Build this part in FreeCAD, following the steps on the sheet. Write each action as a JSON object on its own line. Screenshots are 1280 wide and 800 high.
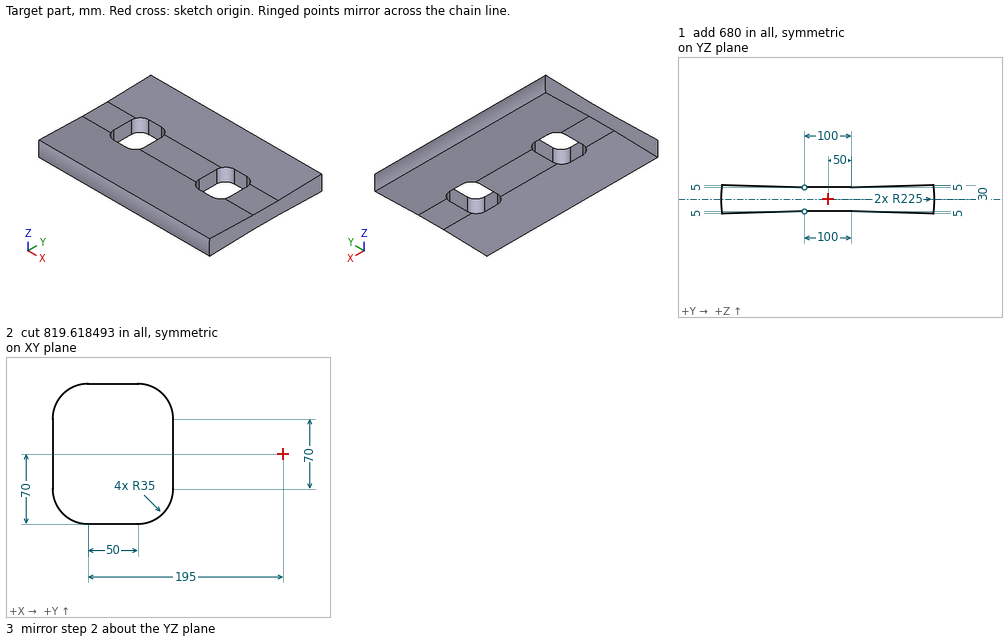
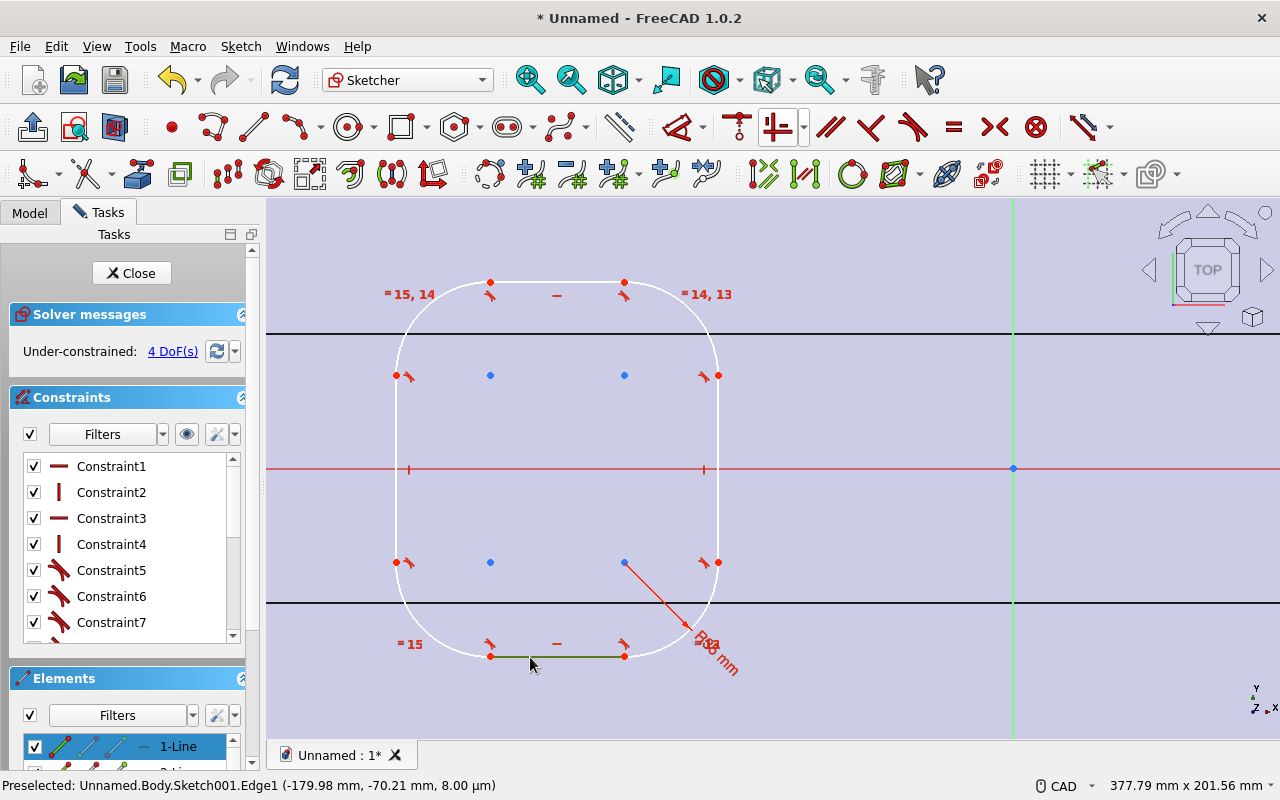
{"action": "key", "text": "l"}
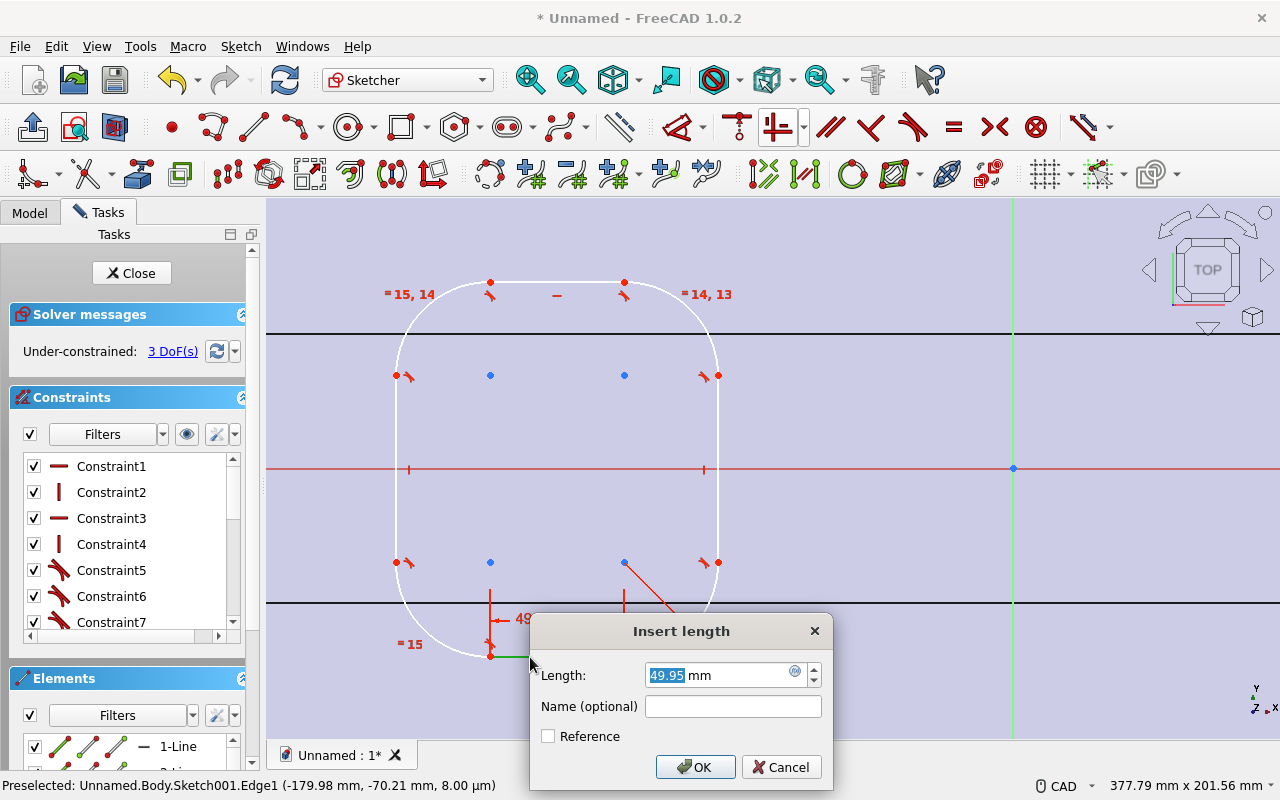
{"action": "type", "text": "50"}
{"action": "key", "text": "Return"}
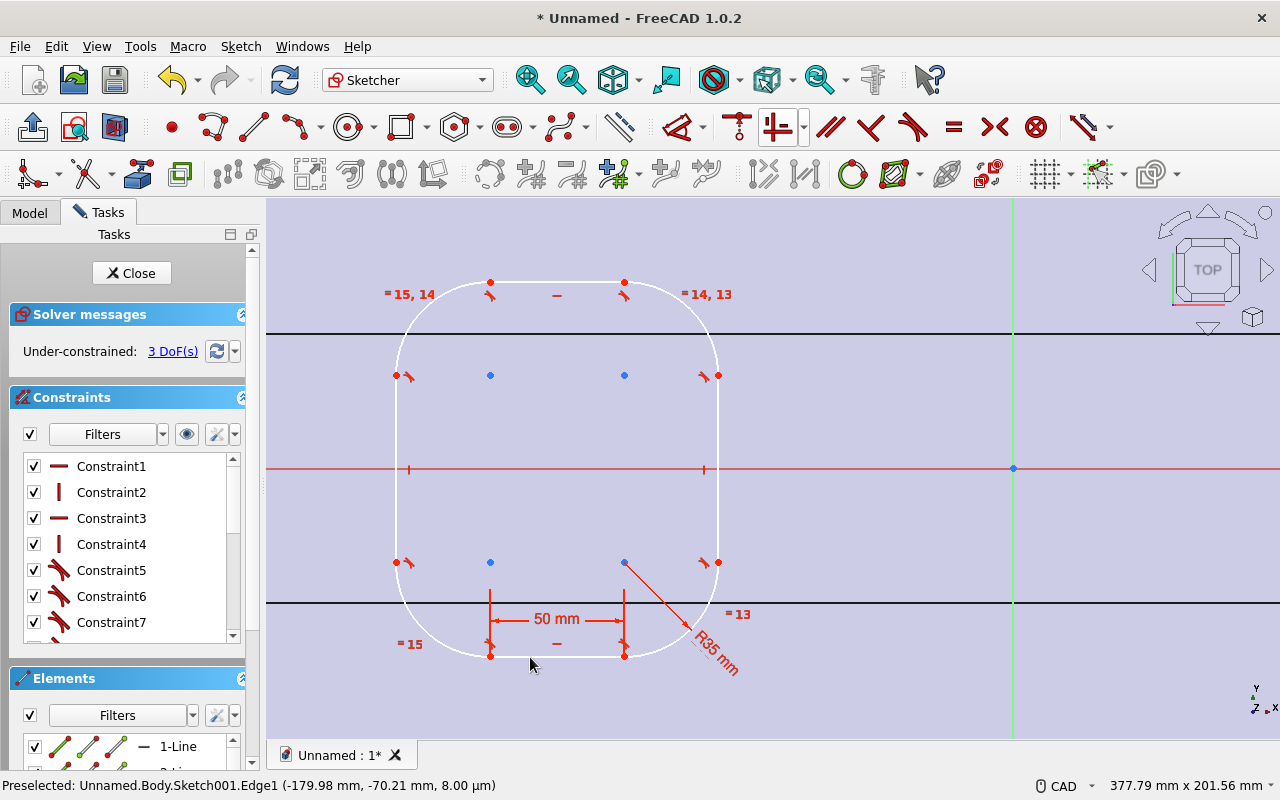
{"action": "left_click", "coordinate": [718, 507]}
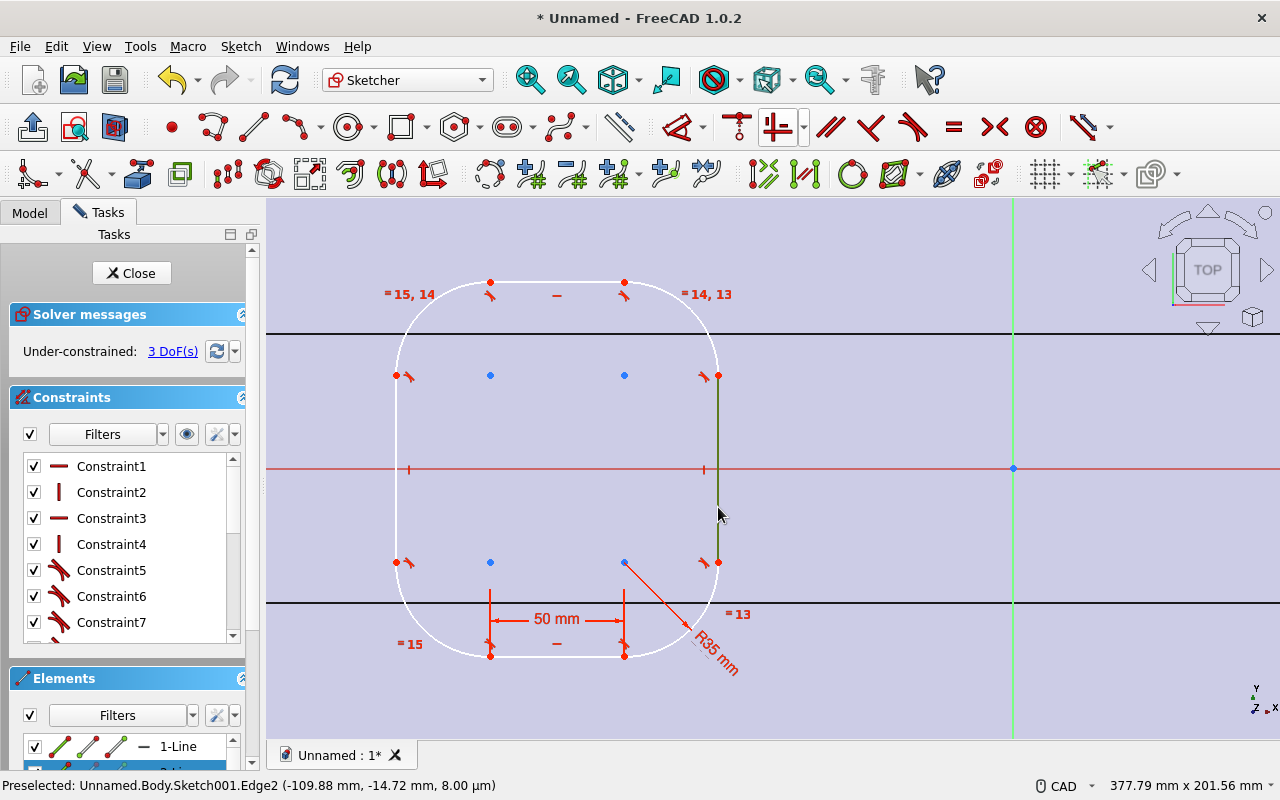
{"action": "key", "text": "i"}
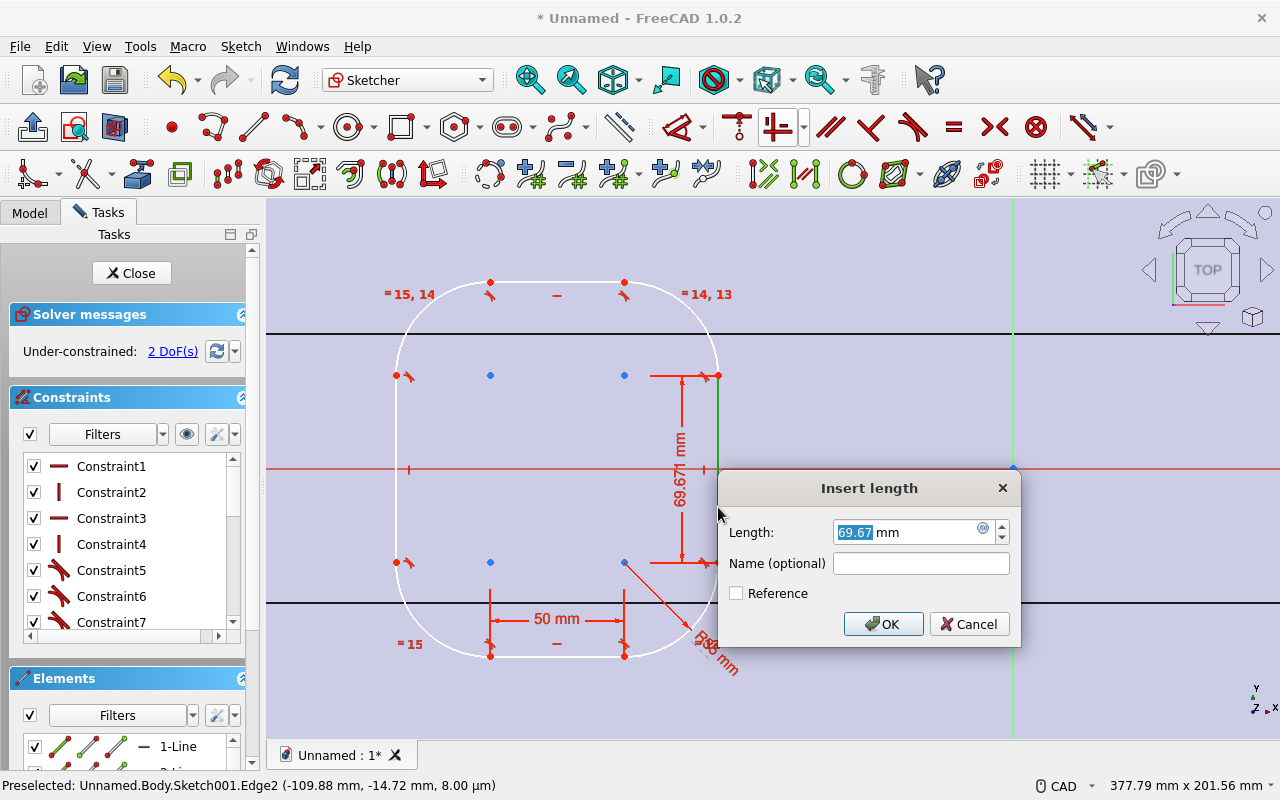
{"action": "type", "text": "70"}
{"action": "key", "text": "Return"}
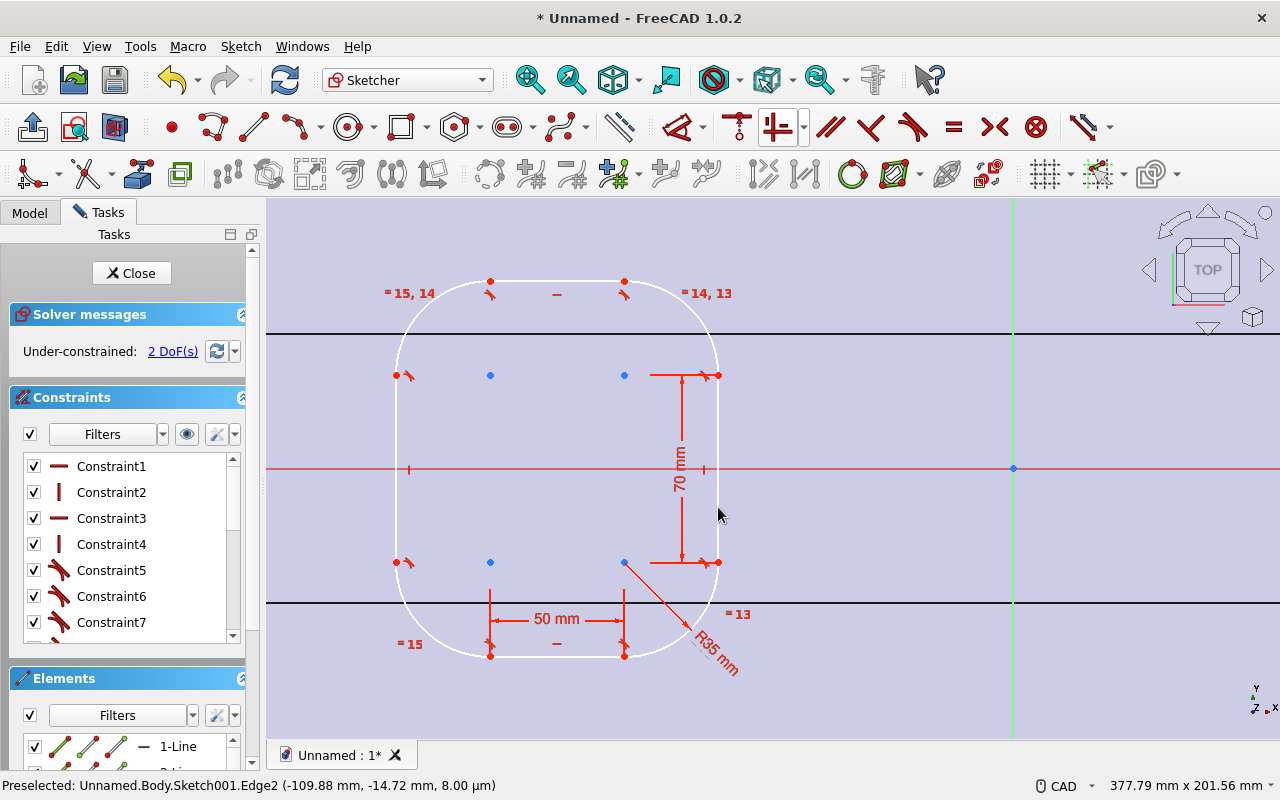
{"action": "left_click", "coordinate": [490, 657]}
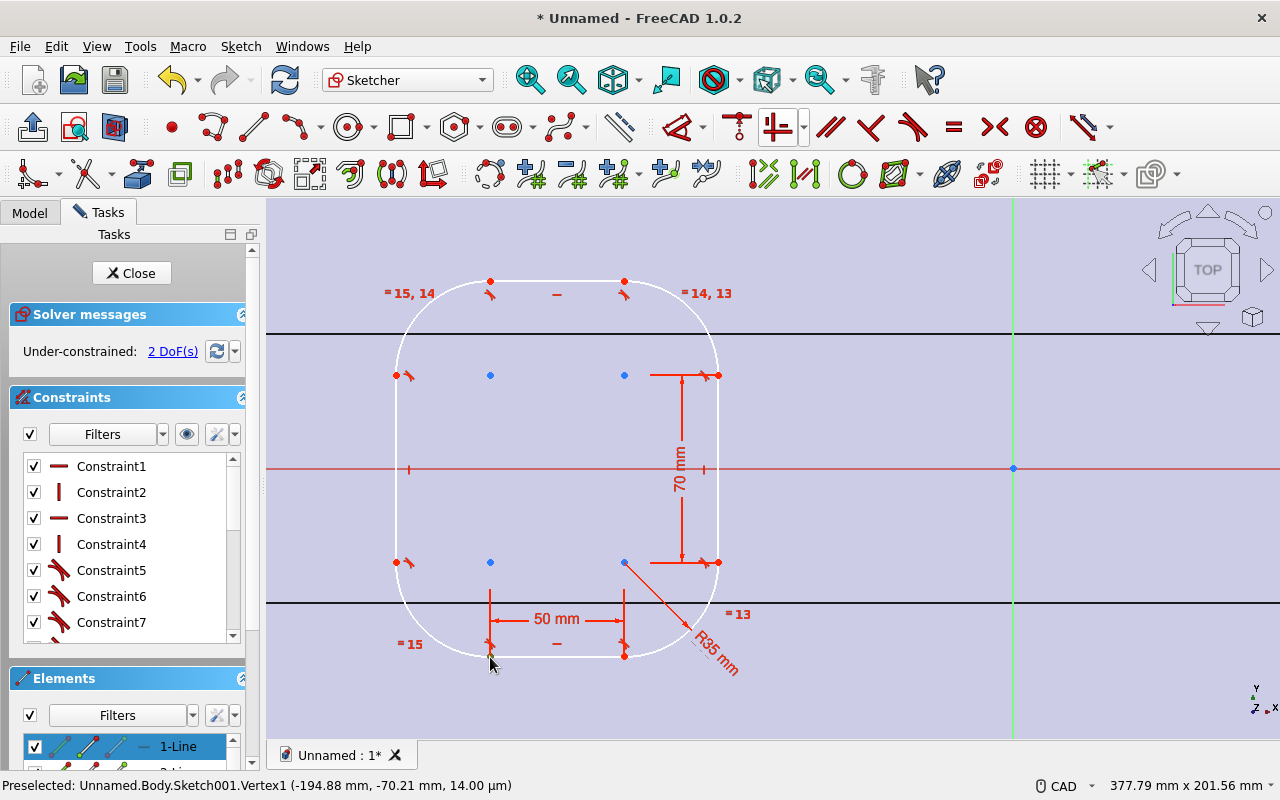
{"action": "key", "text": "i"}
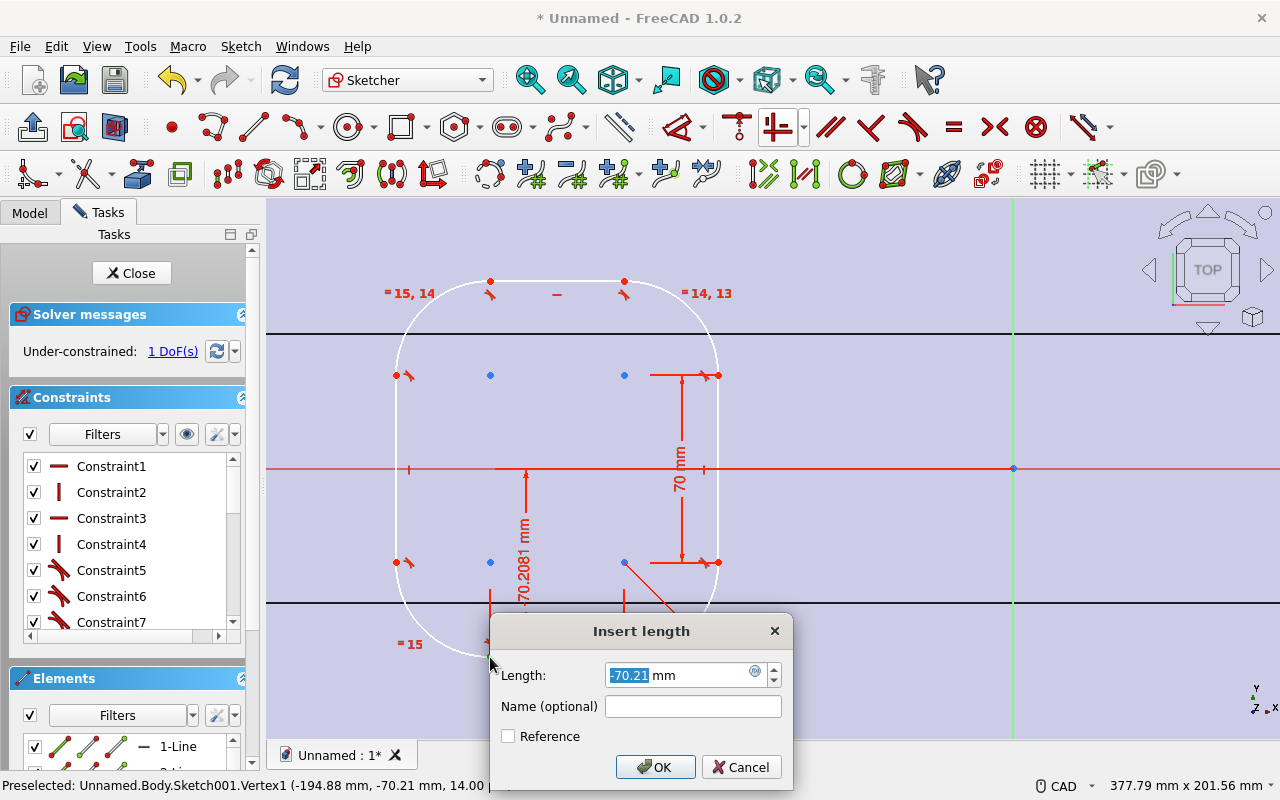
{"action": "type", "text": "-70"}
{"action": "key", "text": "Return"}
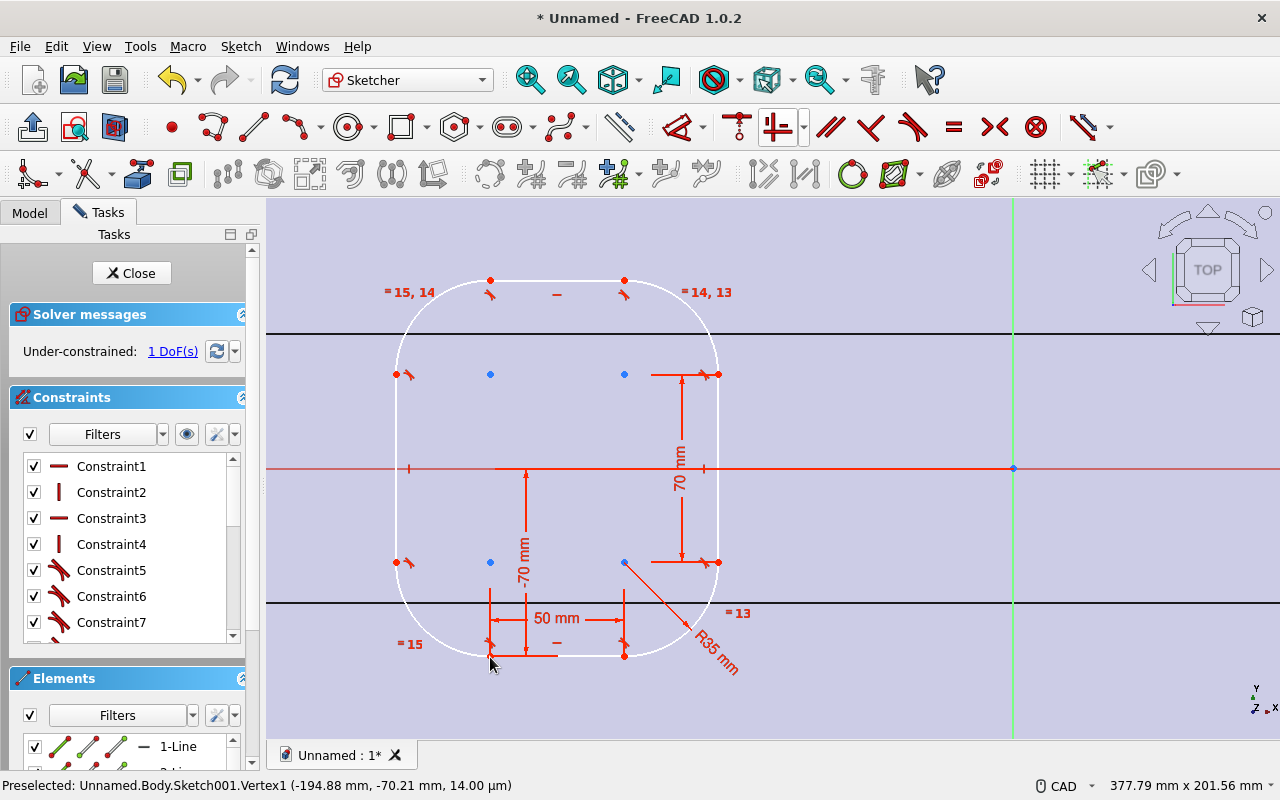
{"action": "left_click", "coordinate": [490, 656]}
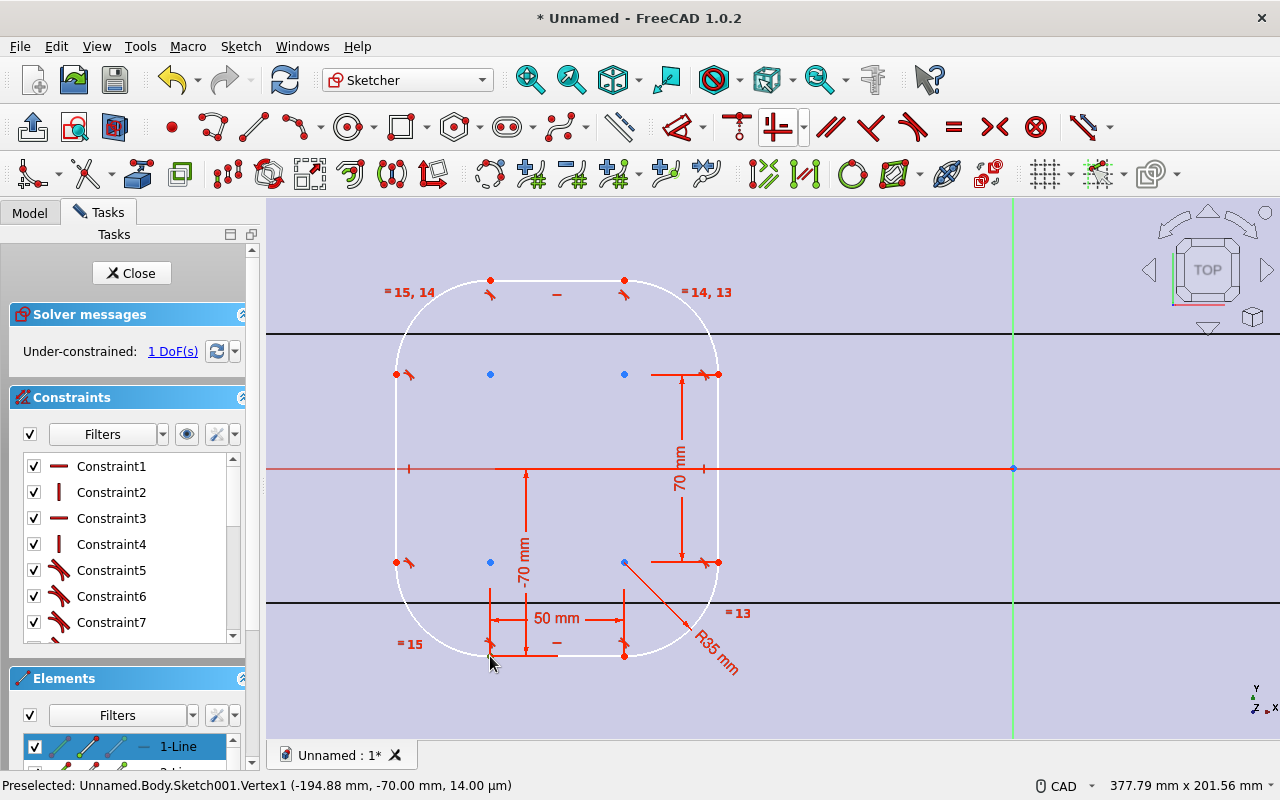
{"action": "key", "text": "l"}